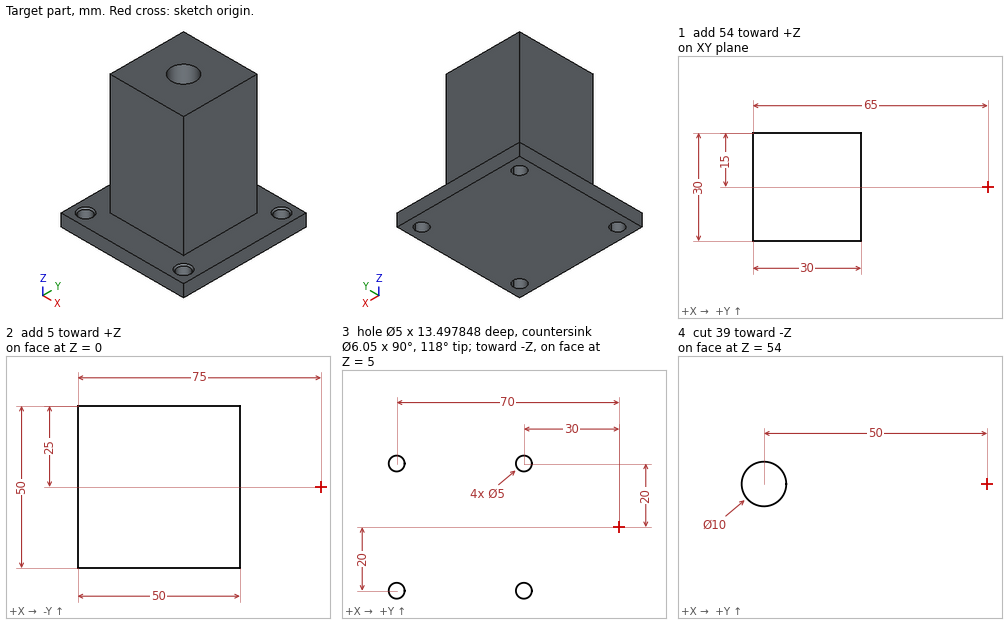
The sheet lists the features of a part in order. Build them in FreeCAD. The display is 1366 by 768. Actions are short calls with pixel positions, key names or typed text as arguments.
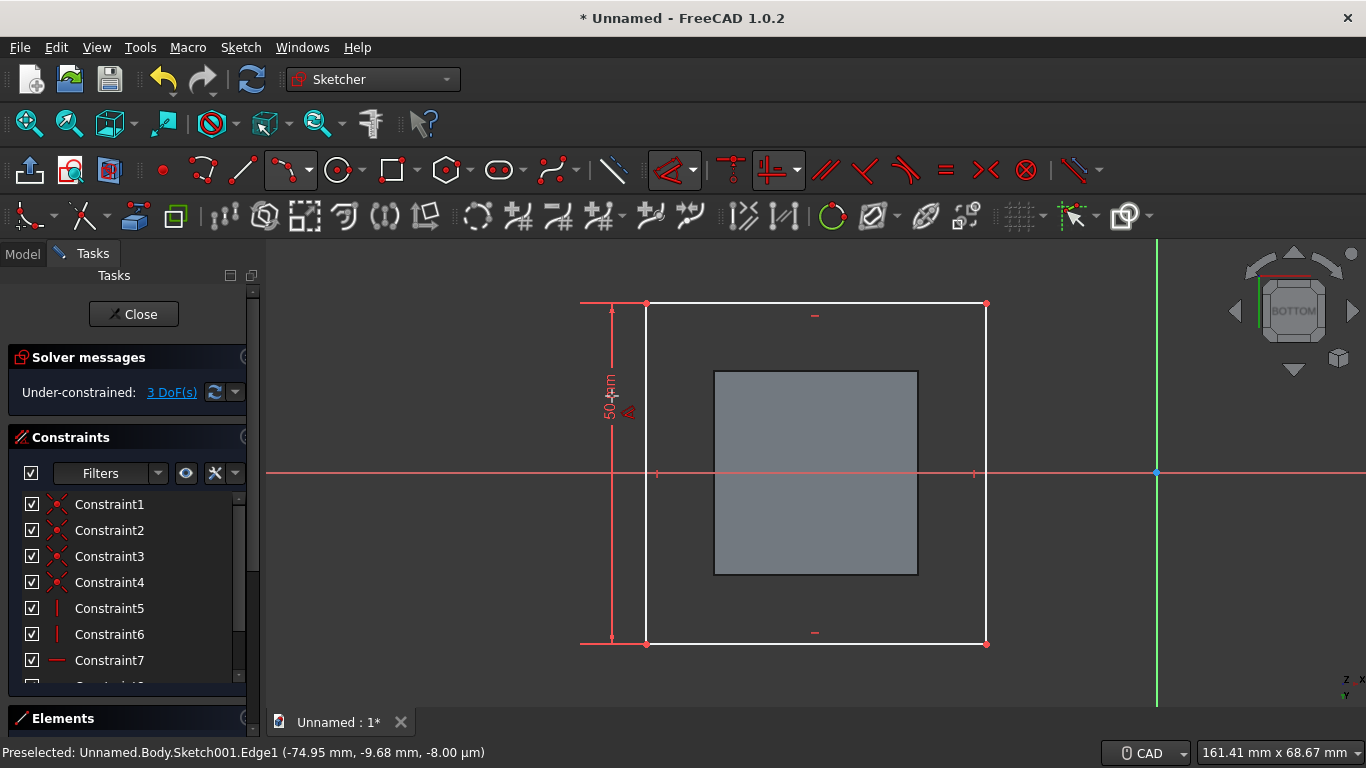
click(748, 644)
click(816, 678)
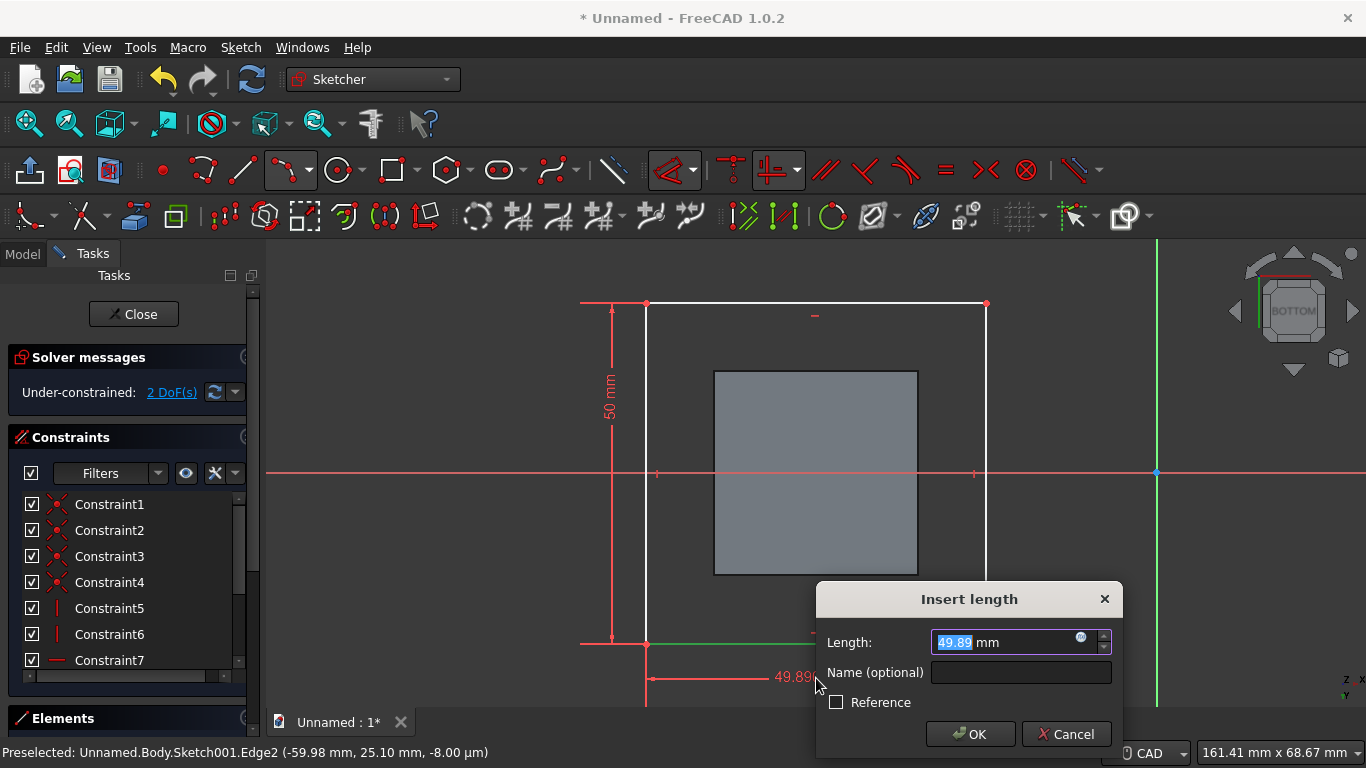
text(50)
key(Return)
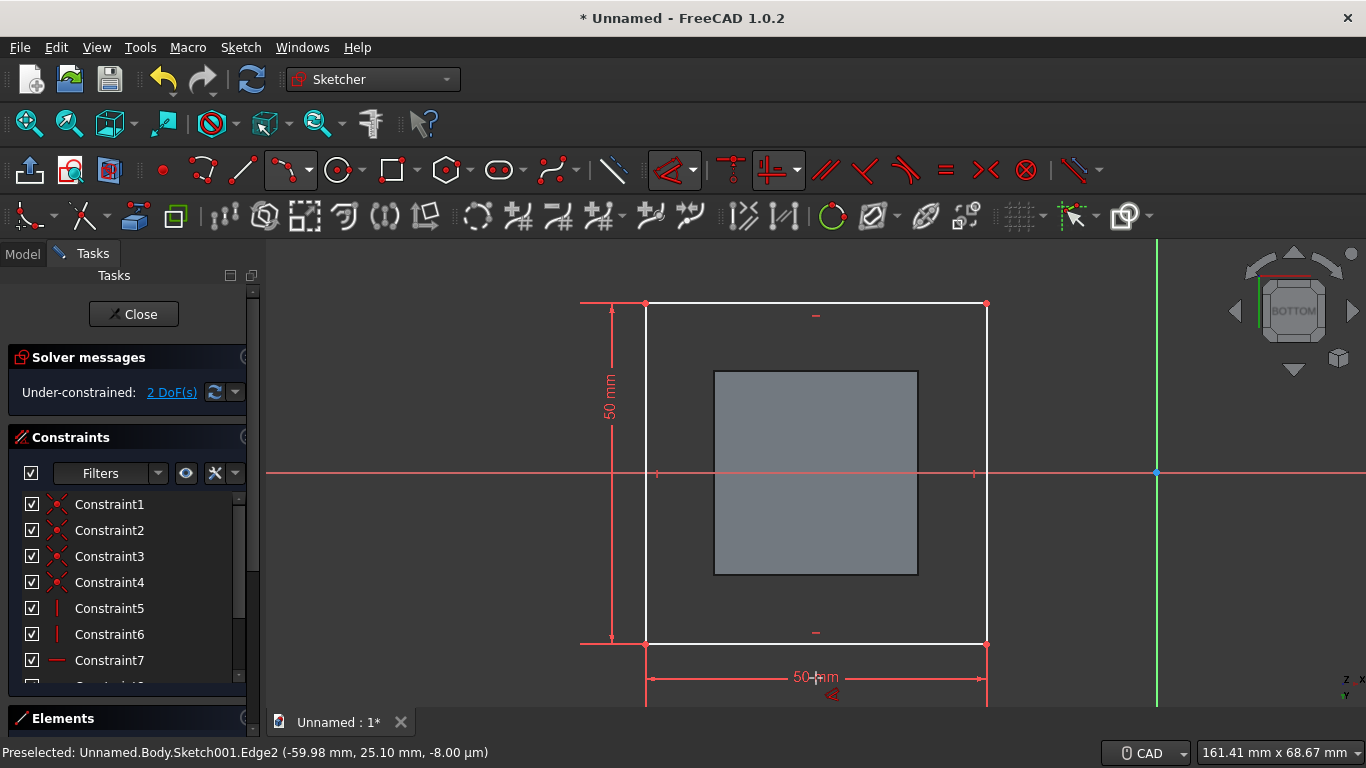
click(646, 303)
click(901, 269)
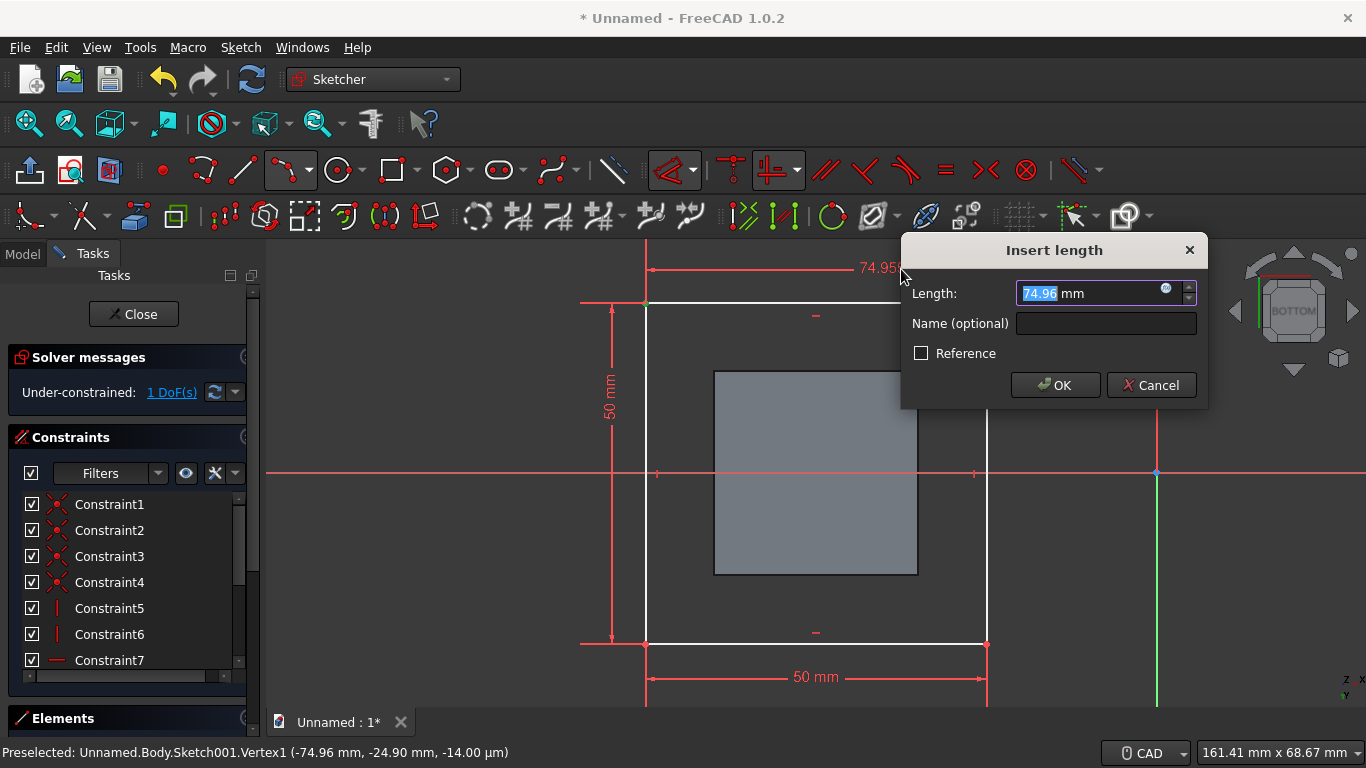
text(75)
key(Return)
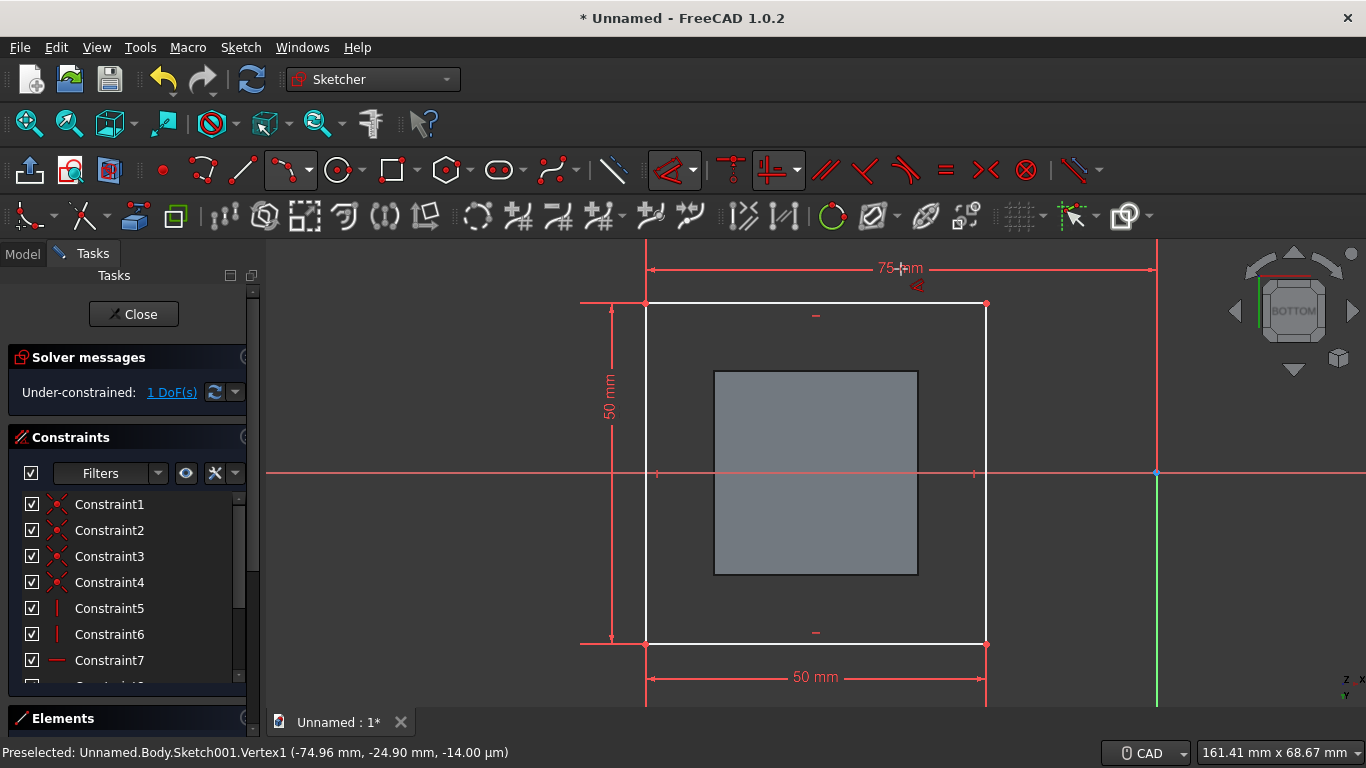
click(646, 303)
click(1191, 388)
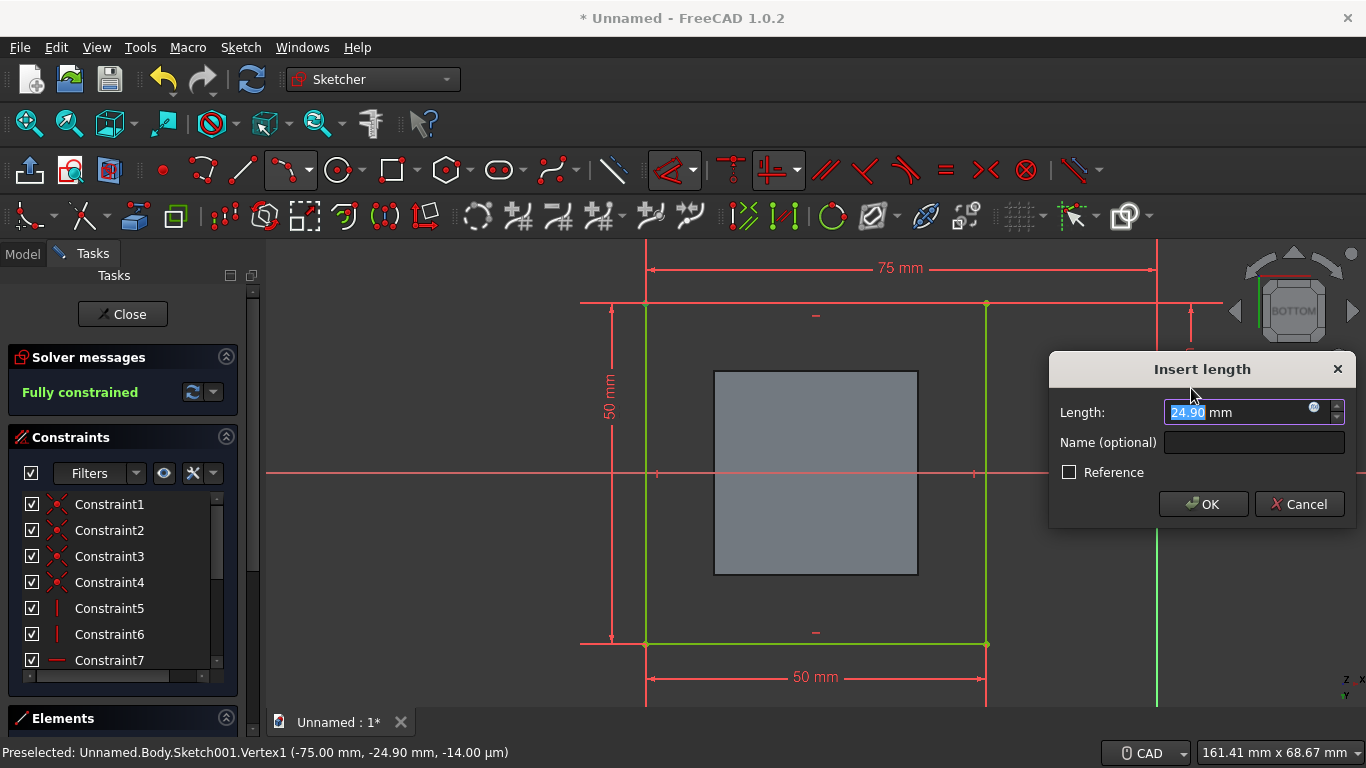
text(25)
key(Return)
key(Escape)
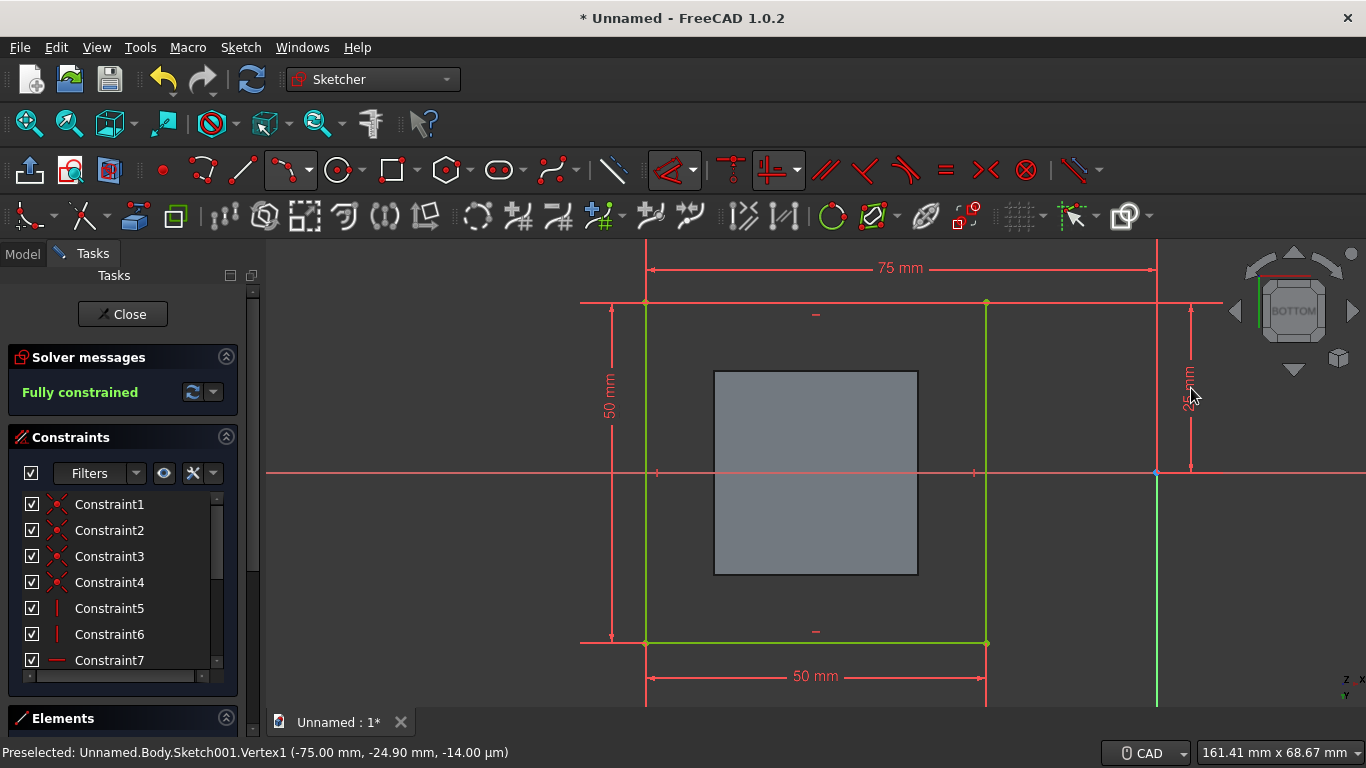
click(123, 314)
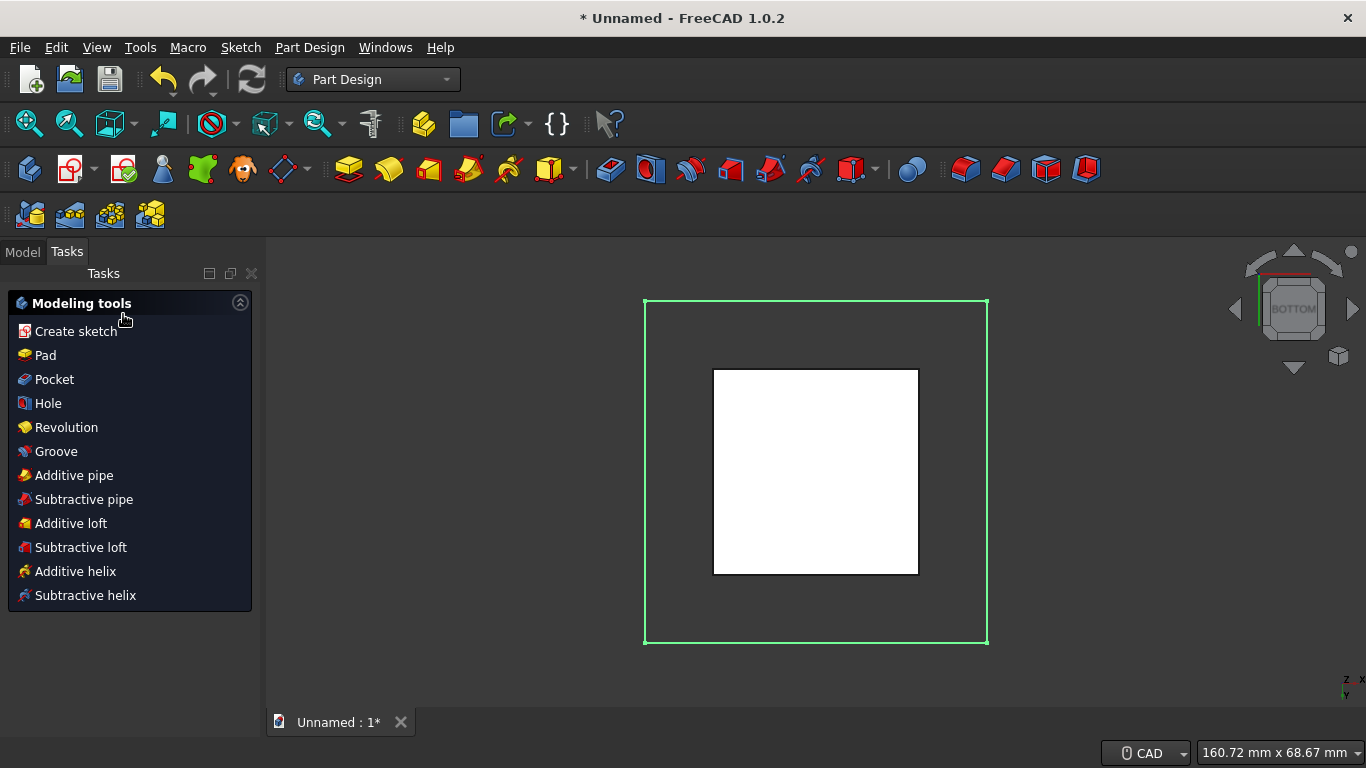
click(350, 170)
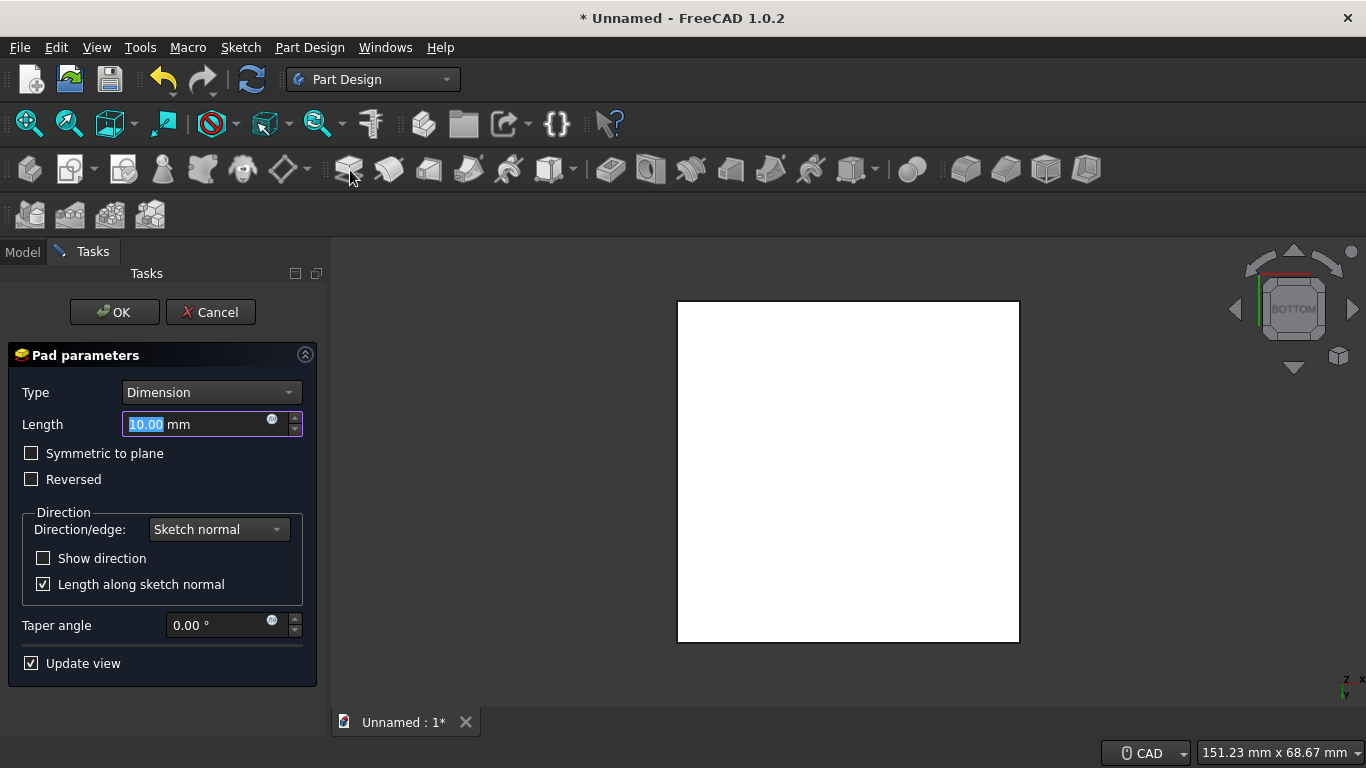
text(5)
key(Tab)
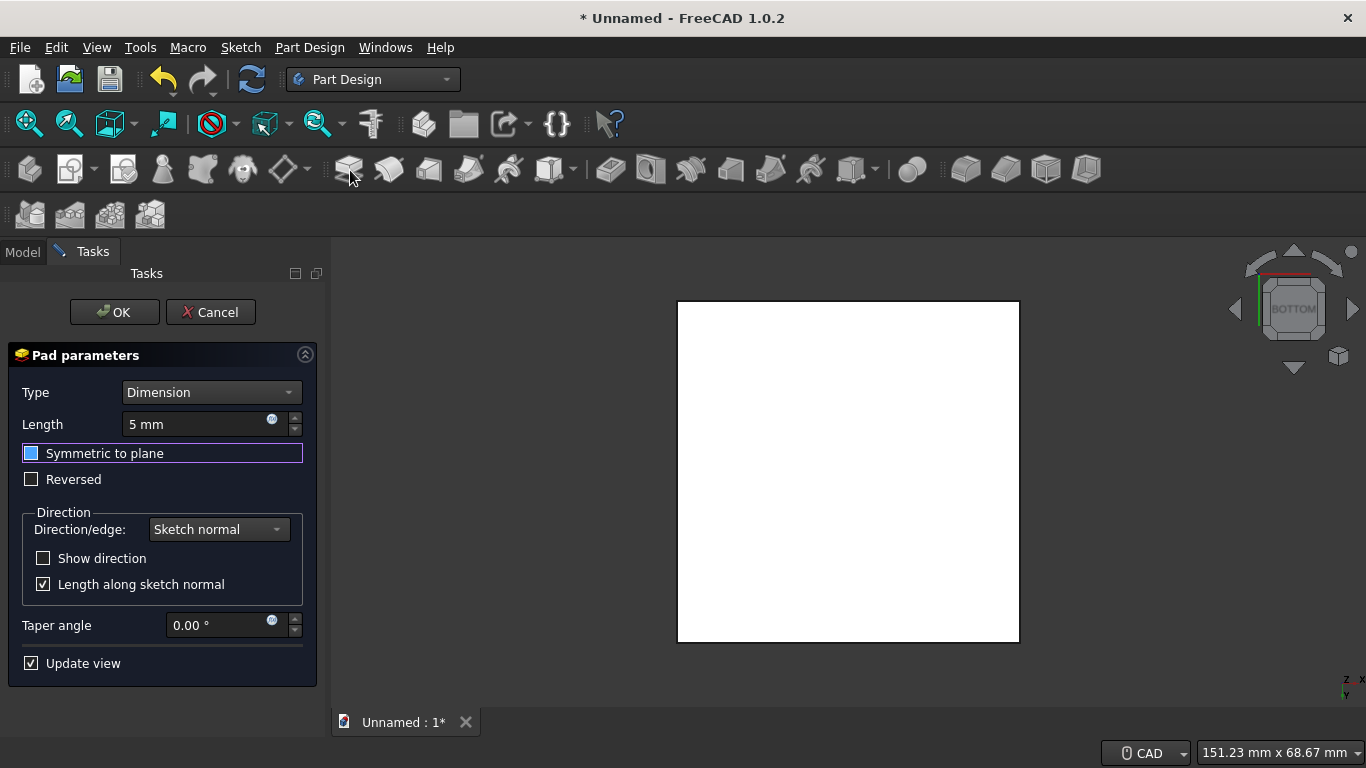
click(30, 479)